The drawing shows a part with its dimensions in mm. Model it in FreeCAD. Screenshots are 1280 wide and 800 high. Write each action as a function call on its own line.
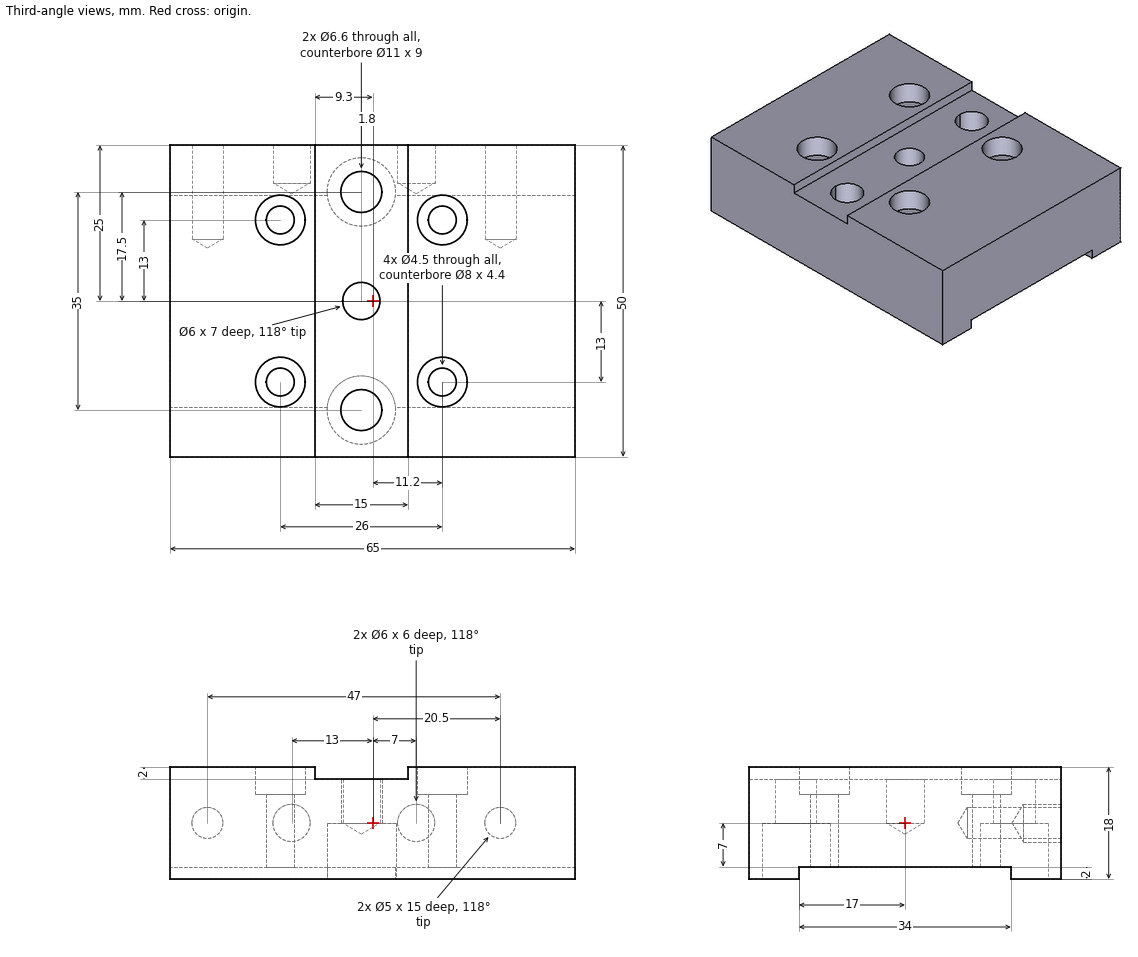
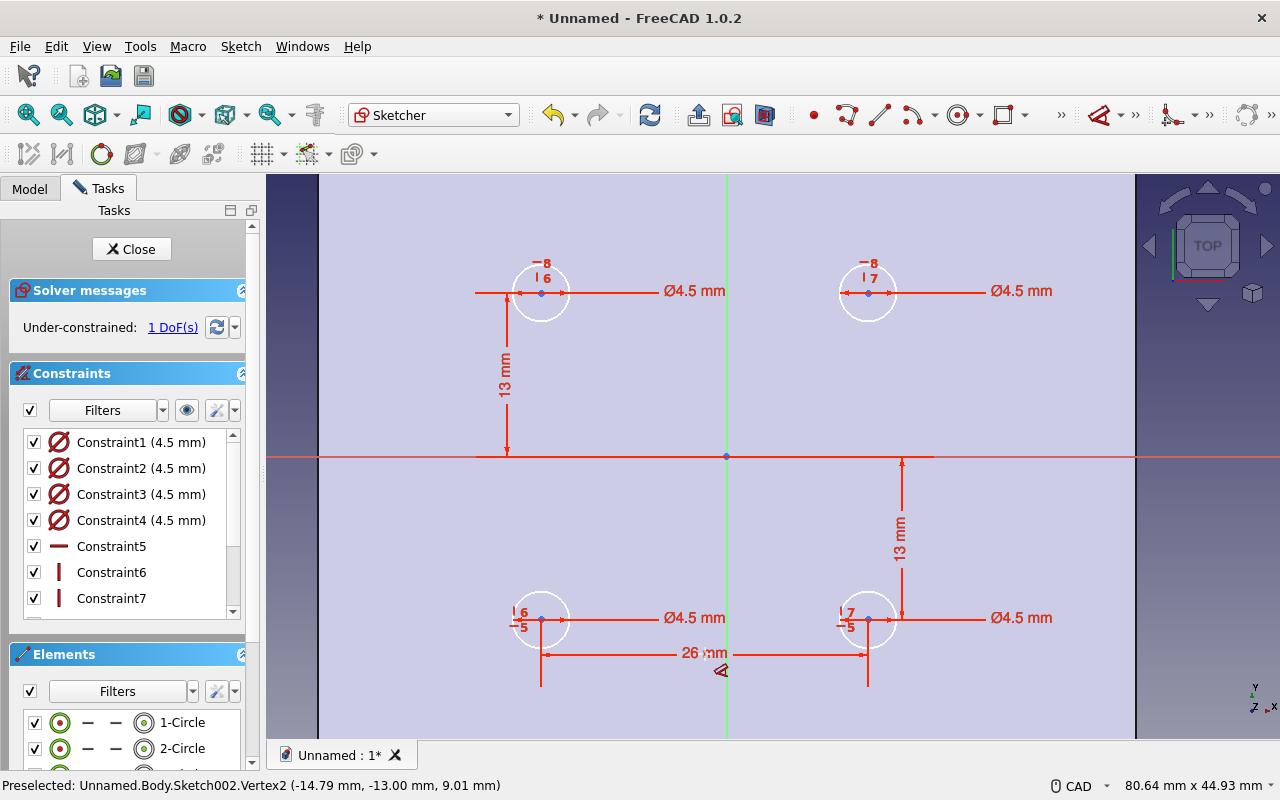
click(868, 620)
click(797, 654)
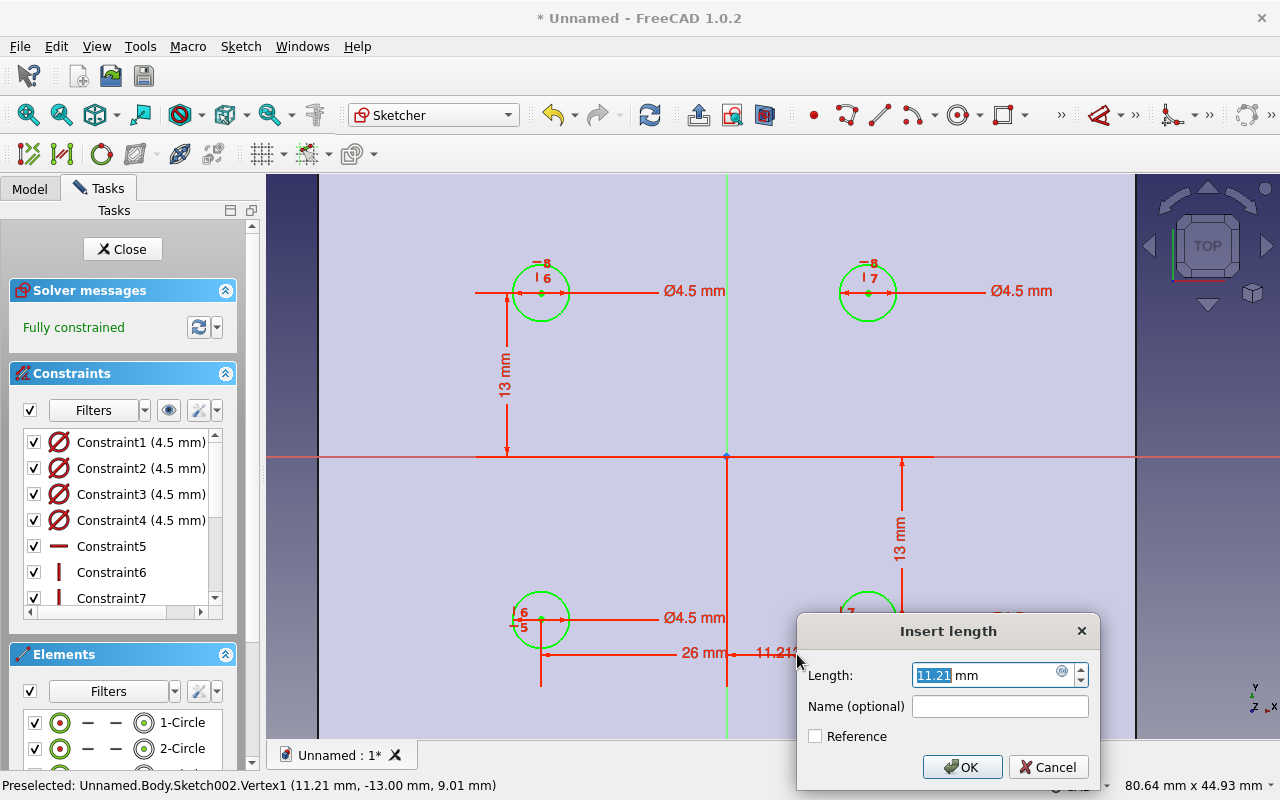
text(11.2)
key(Return)
key(Escape)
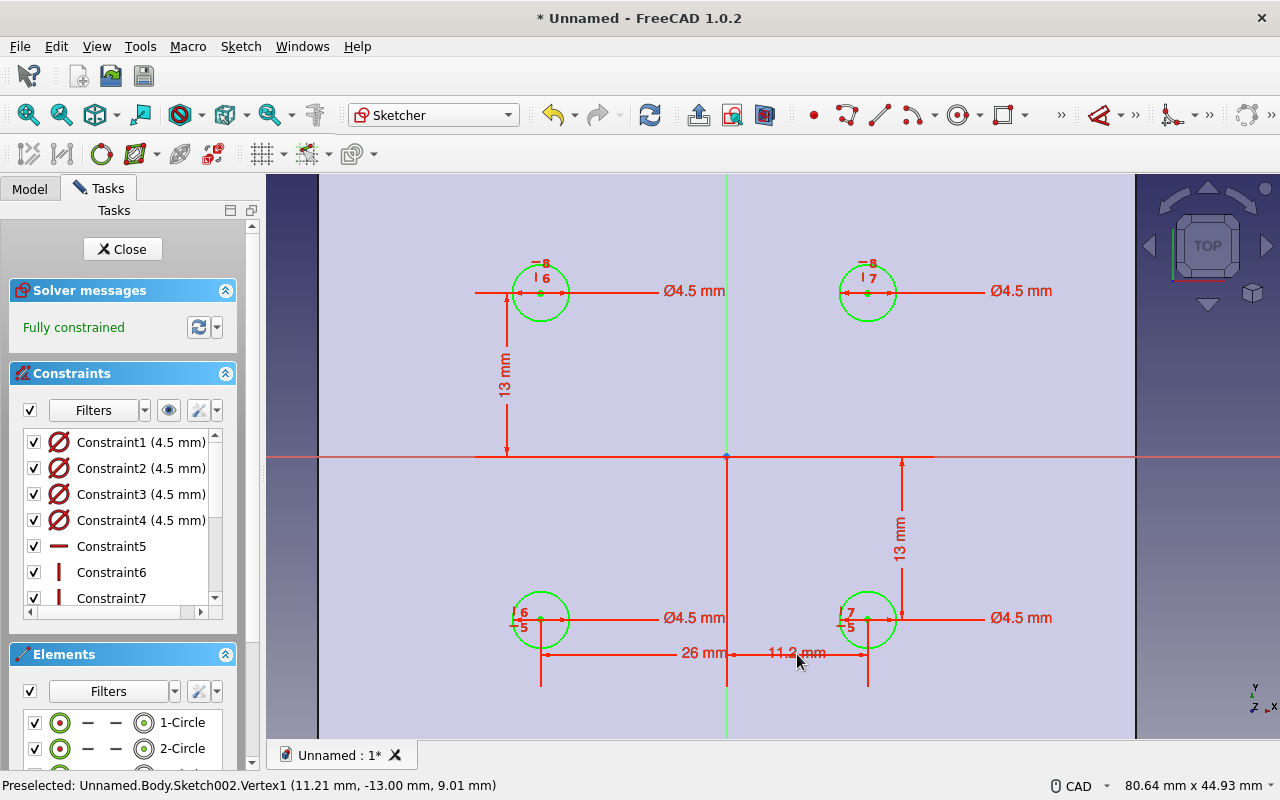
click(123, 249)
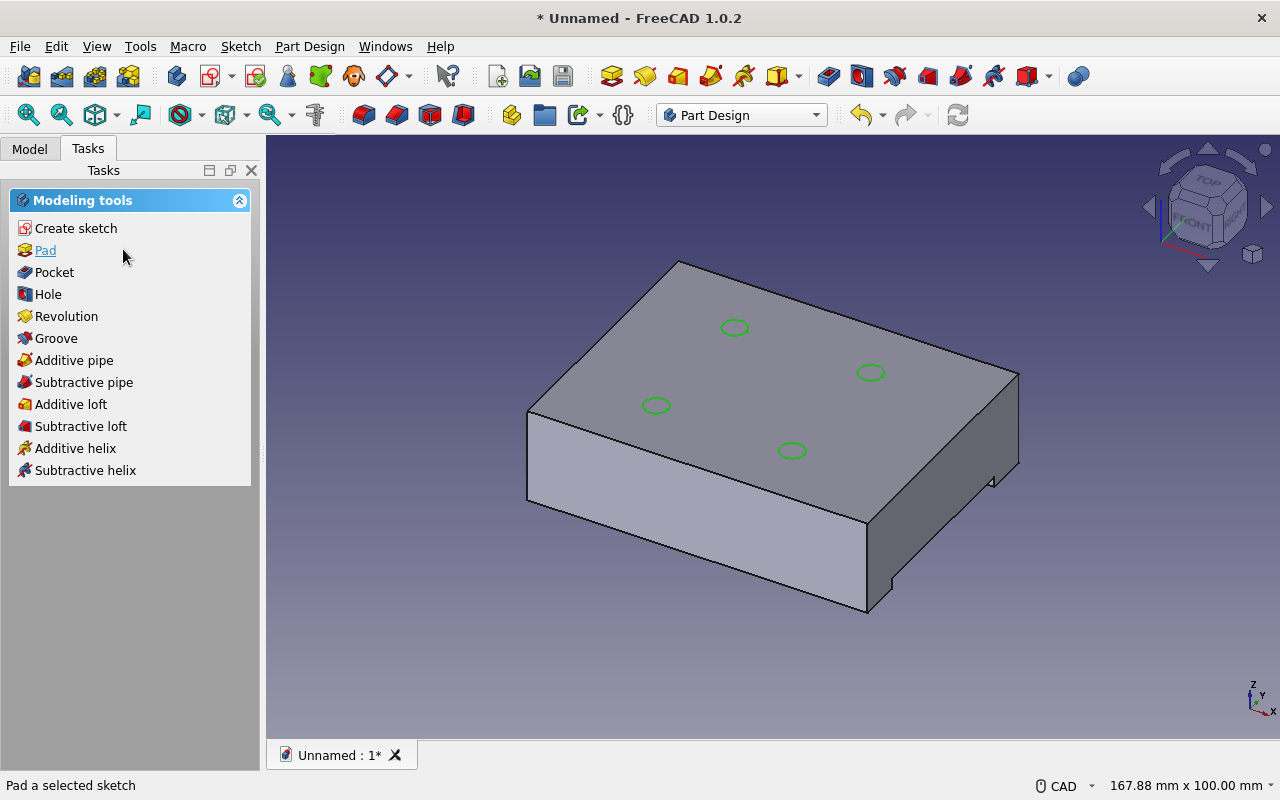
click(862, 76)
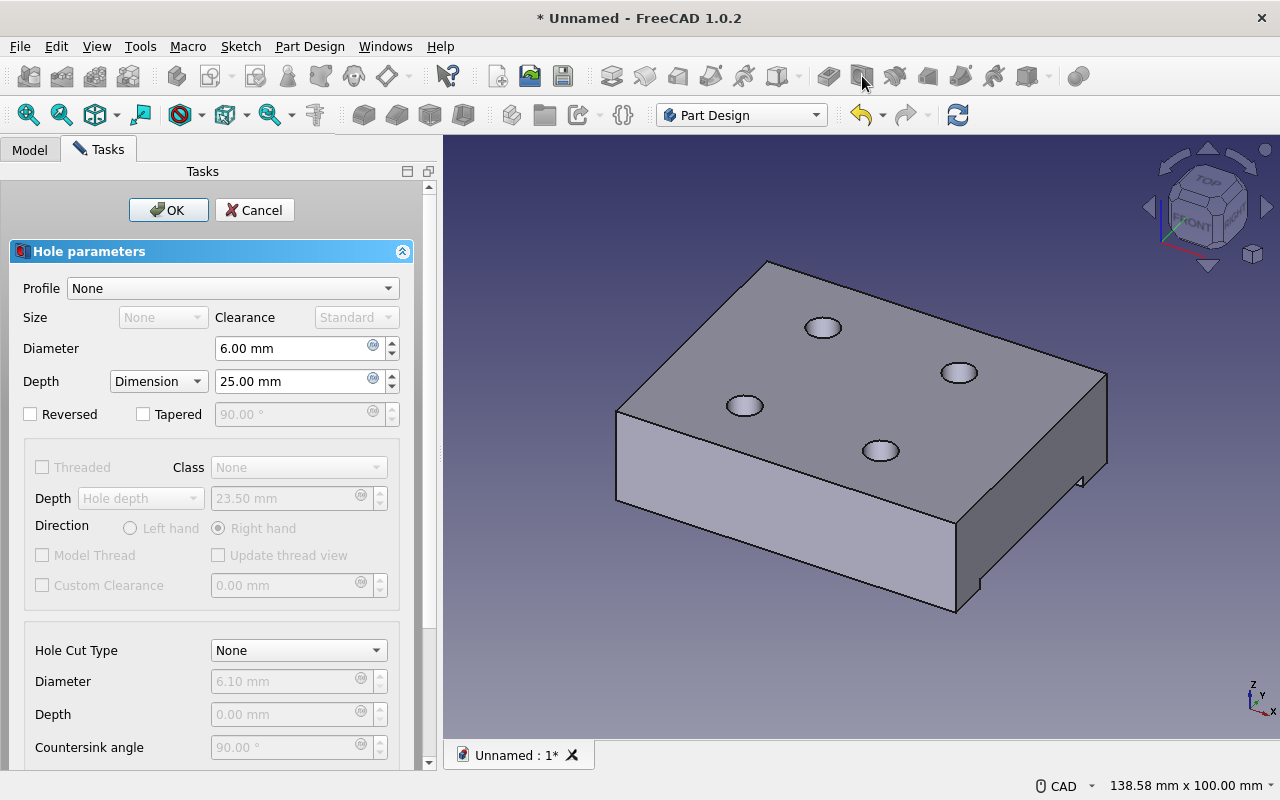
triple_click(300, 348)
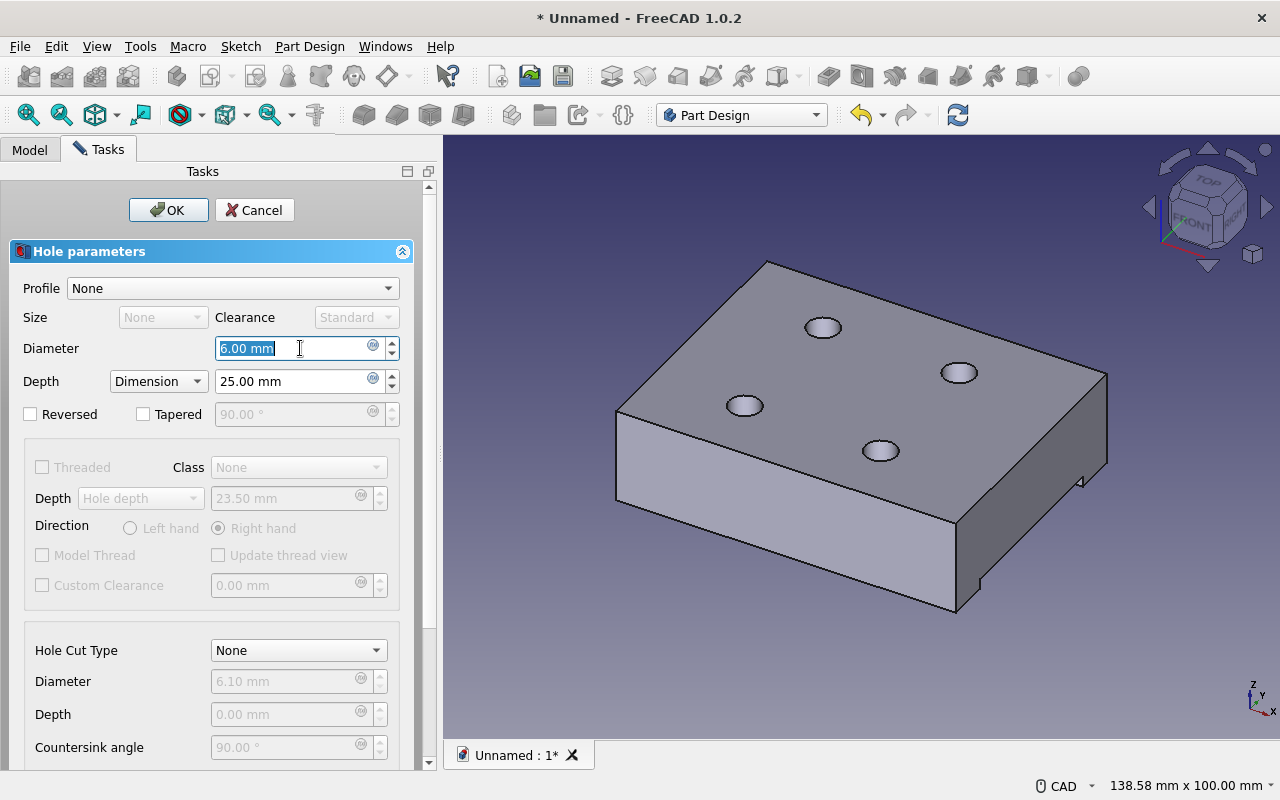
text(4.5)
key(Tab)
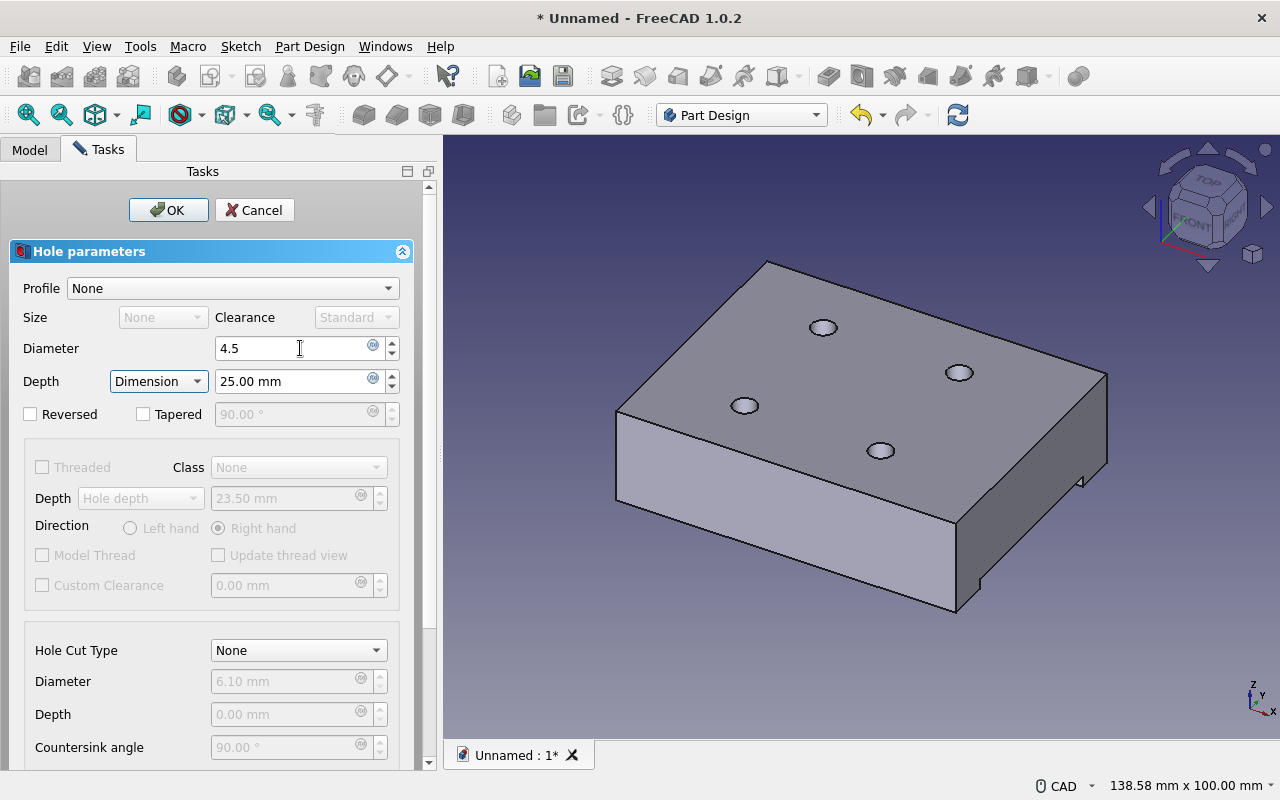
click(160, 382)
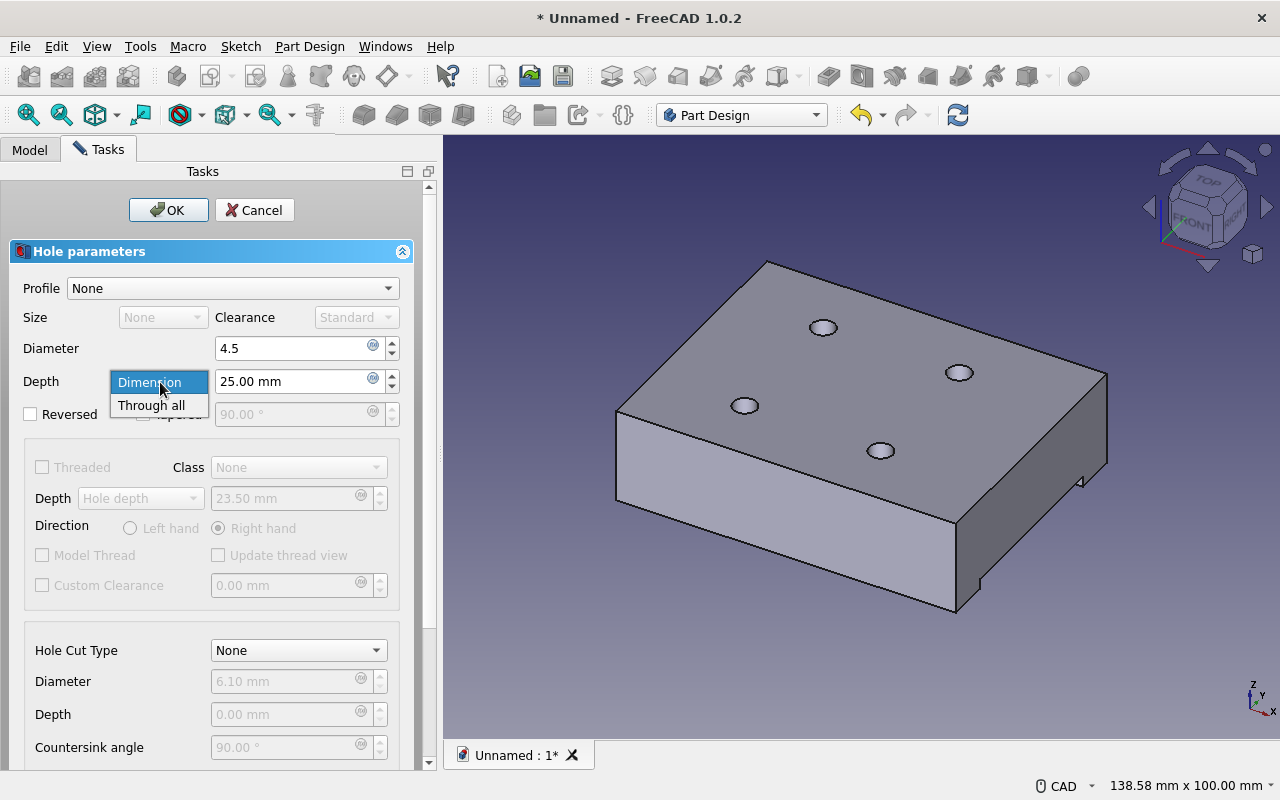
click(158, 406)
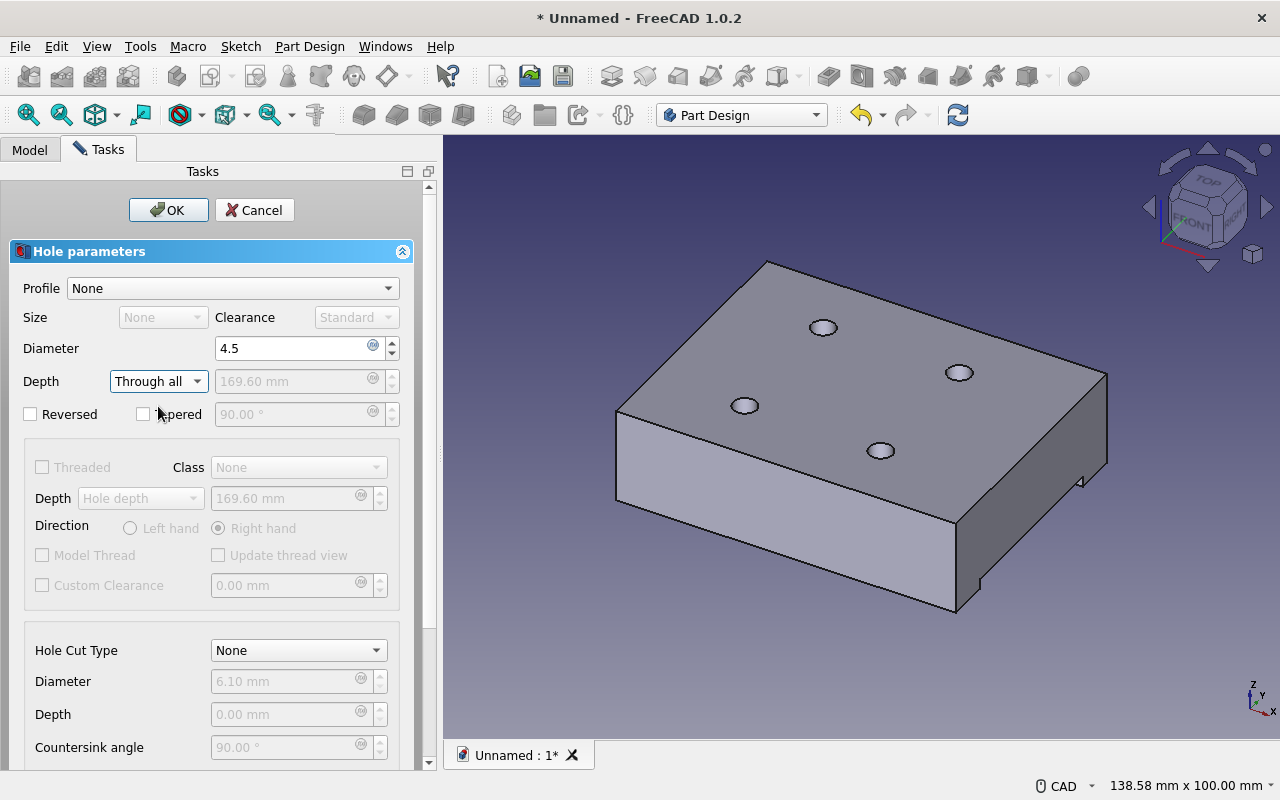
click(300, 650)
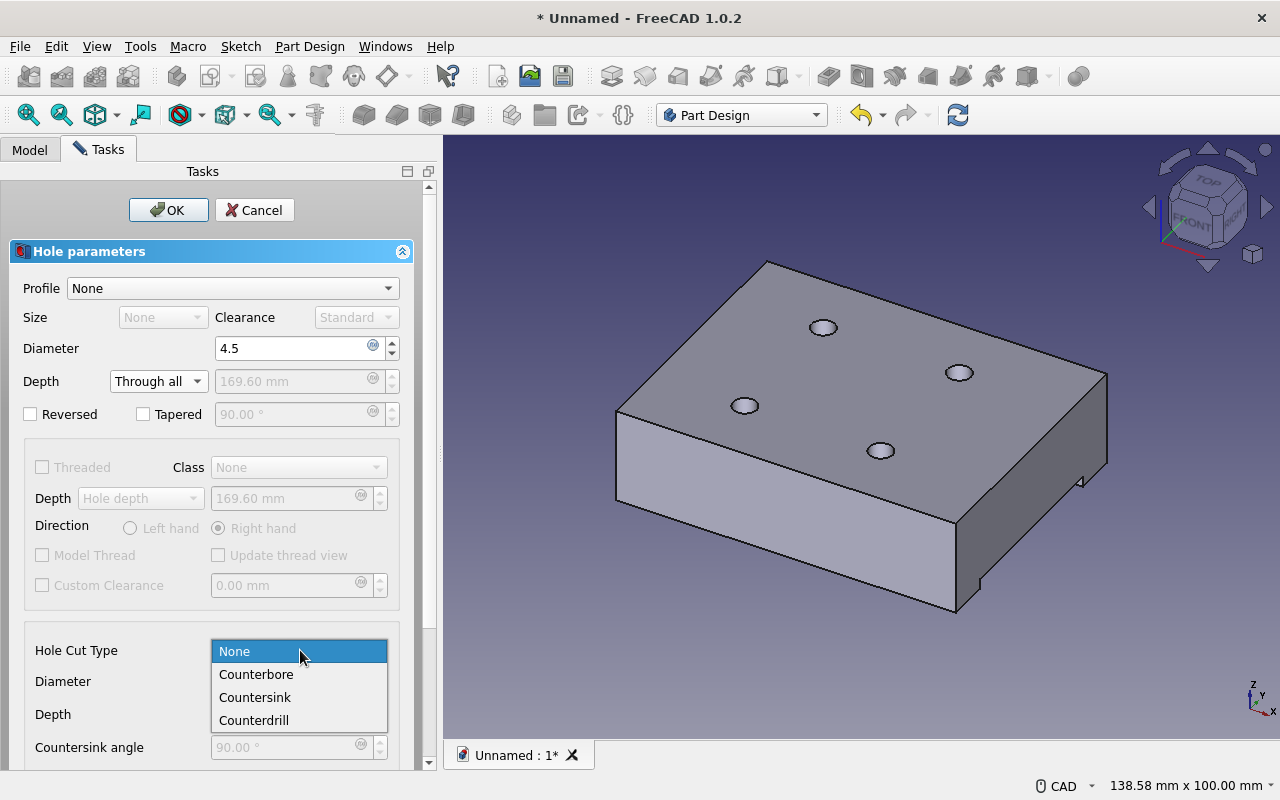
click(298, 674)